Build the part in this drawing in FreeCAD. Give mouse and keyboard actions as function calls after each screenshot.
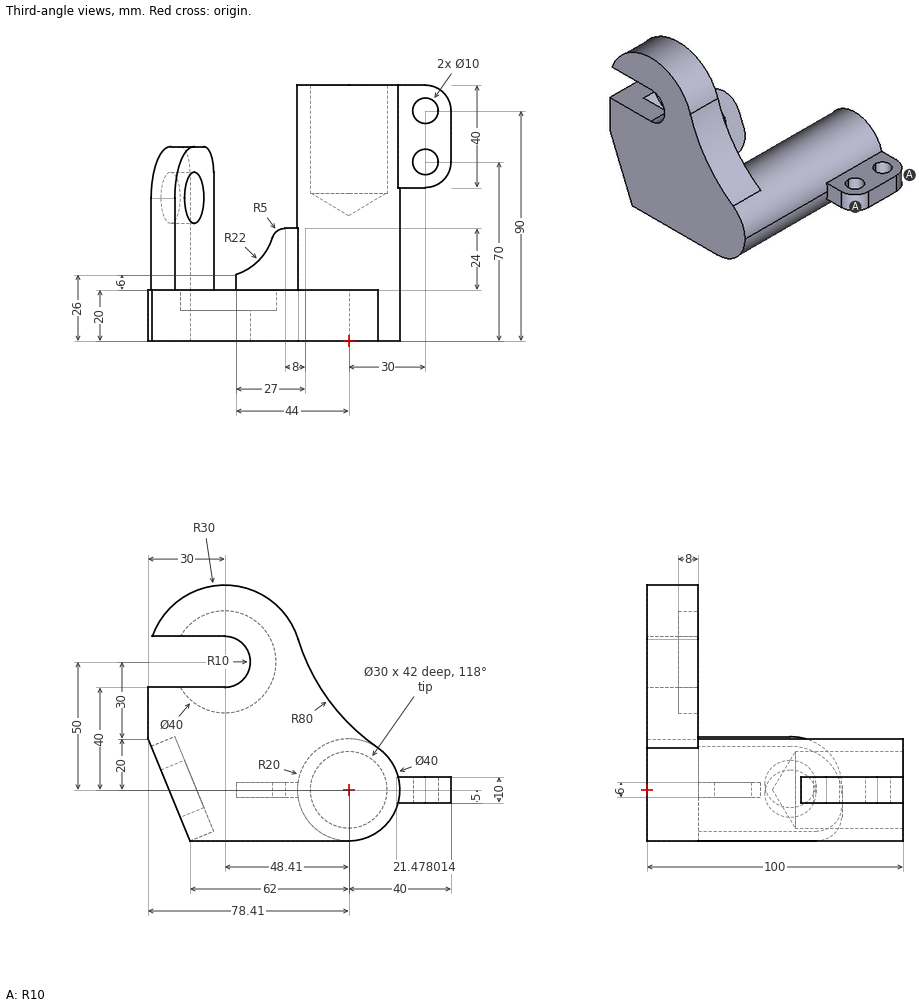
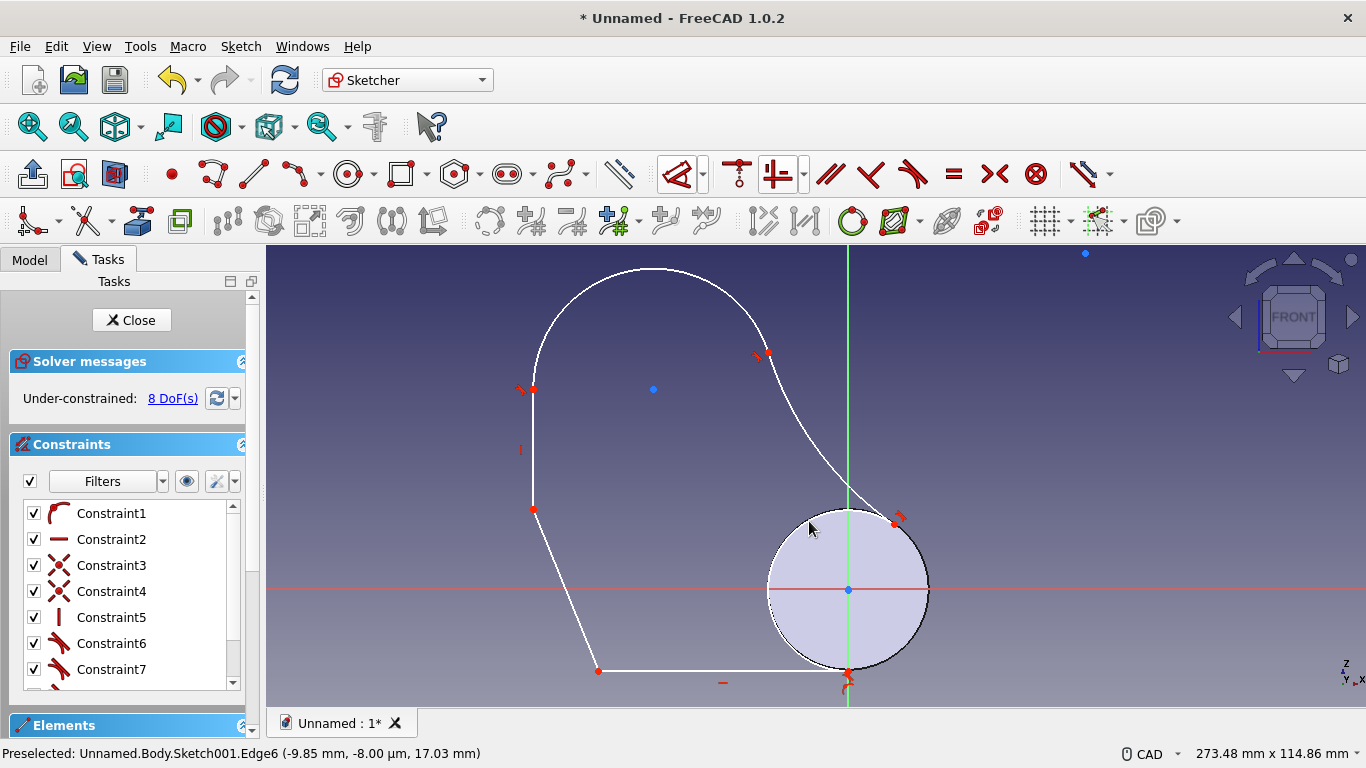
click(848, 591)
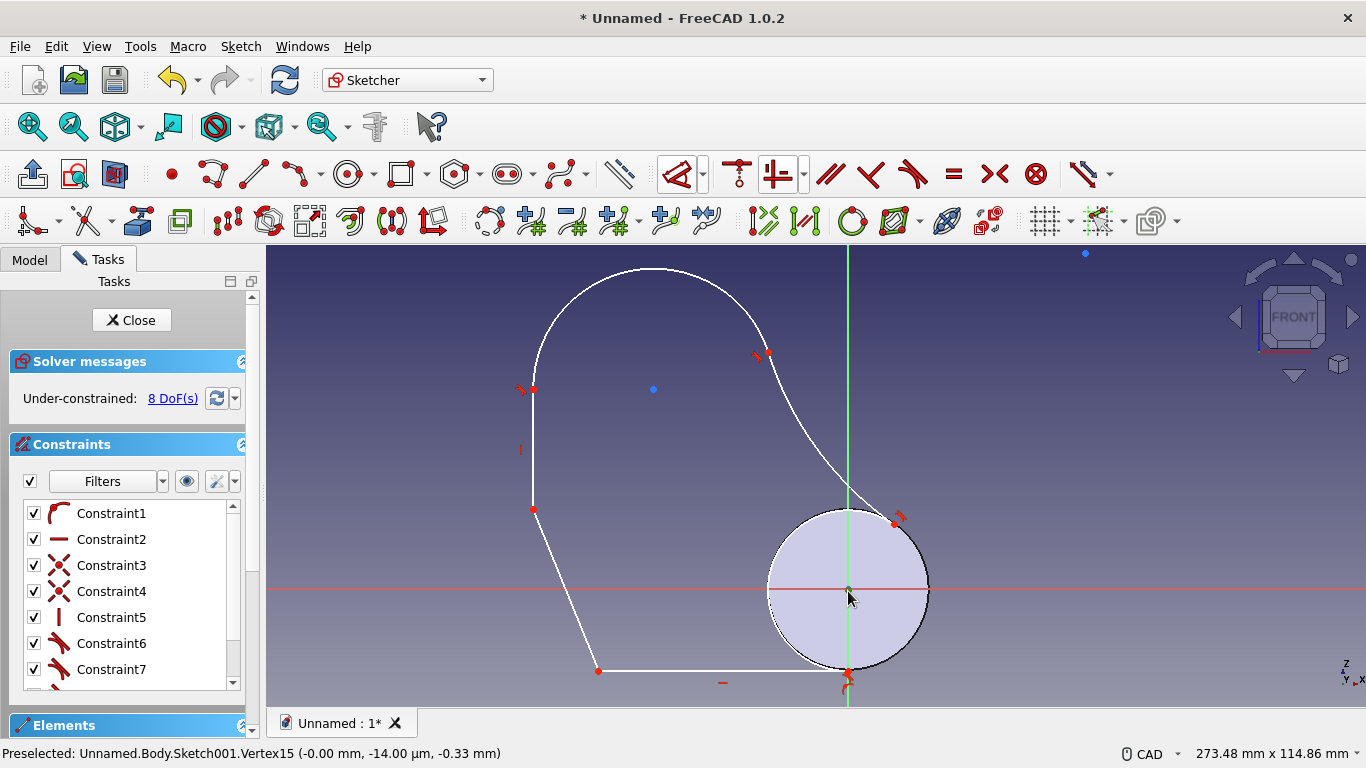
click(359, 589)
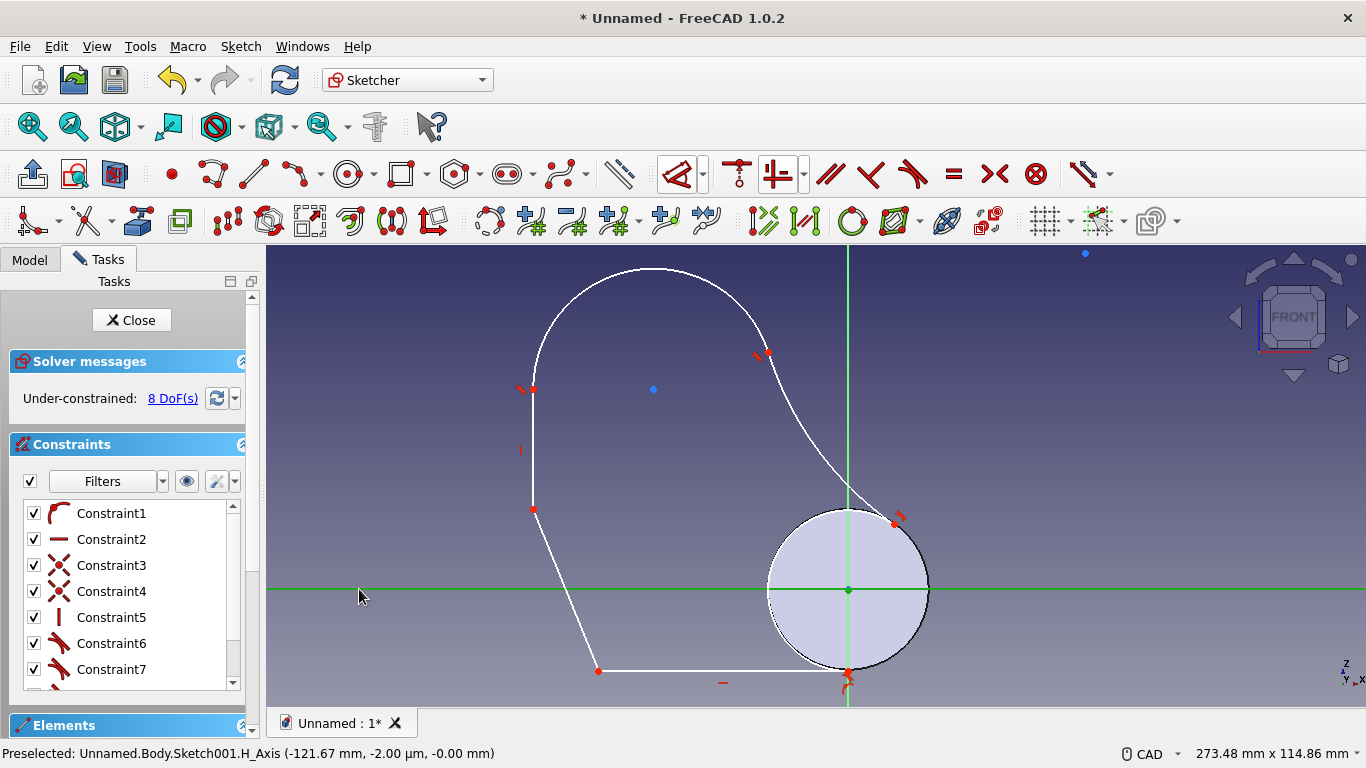
key(c)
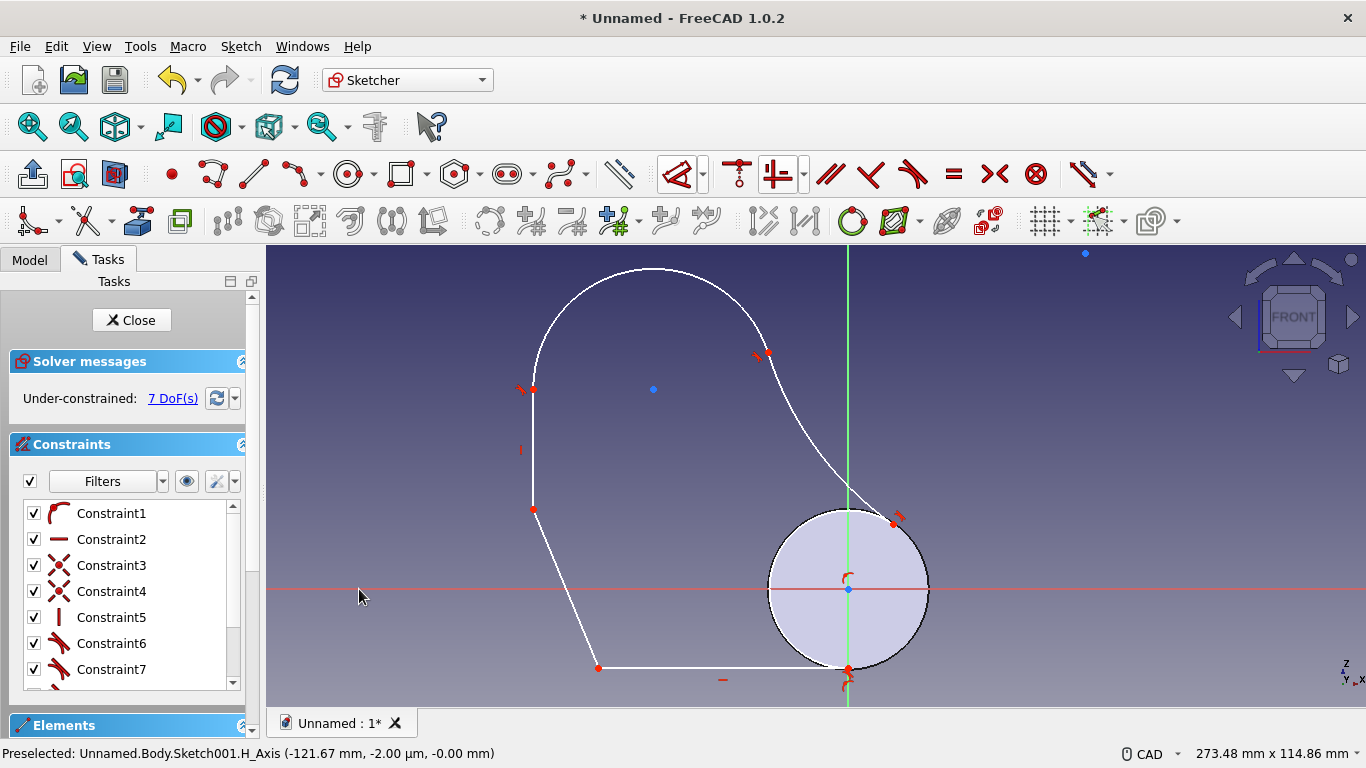
key(d)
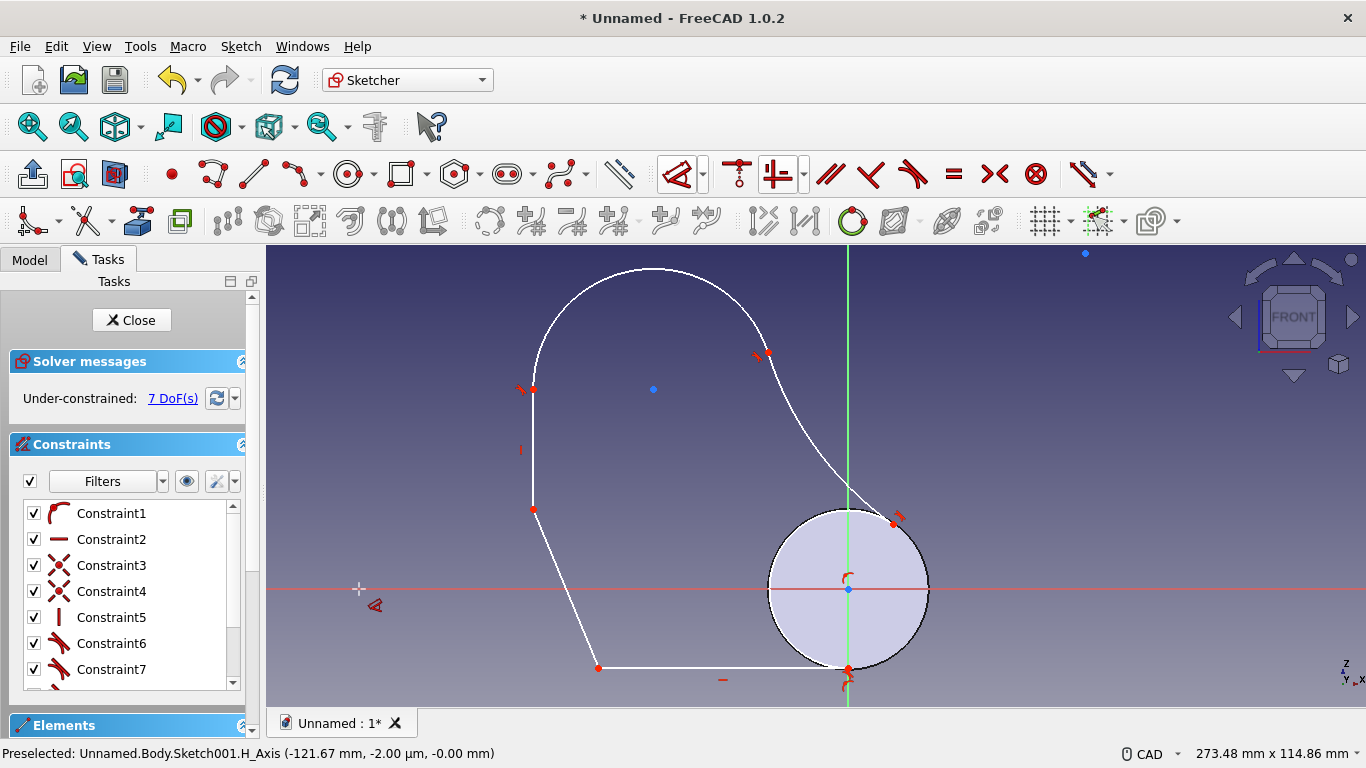
click(702, 279)
click(774, 296)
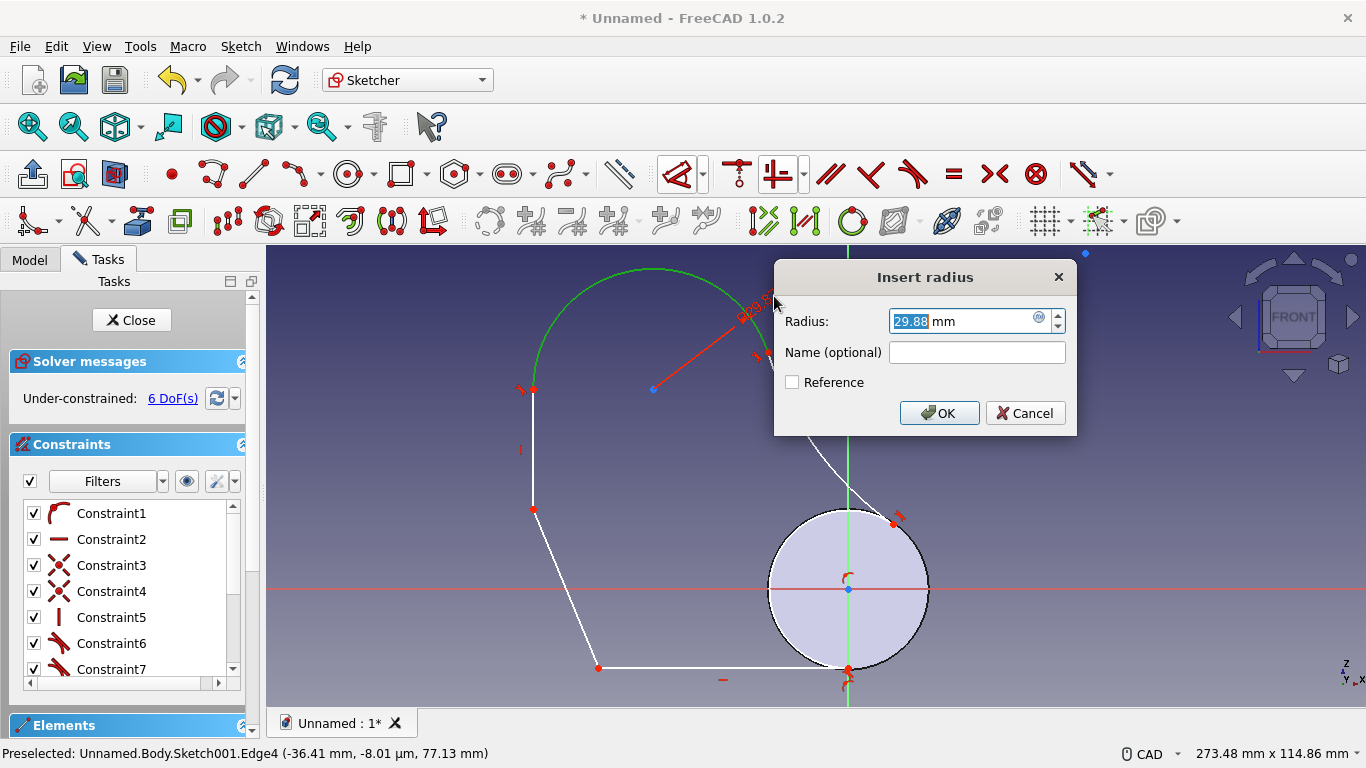
text(30)
key(Return)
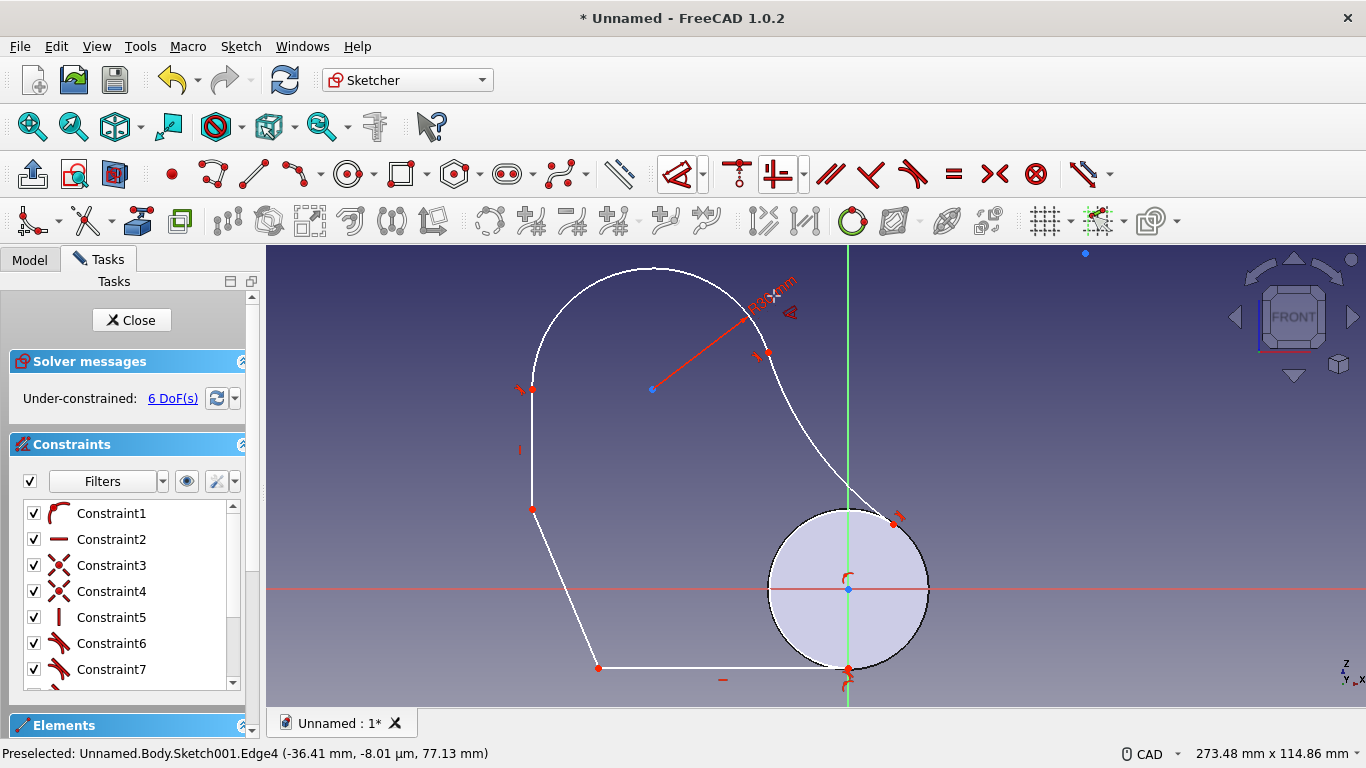
click(794, 413)
click(766, 428)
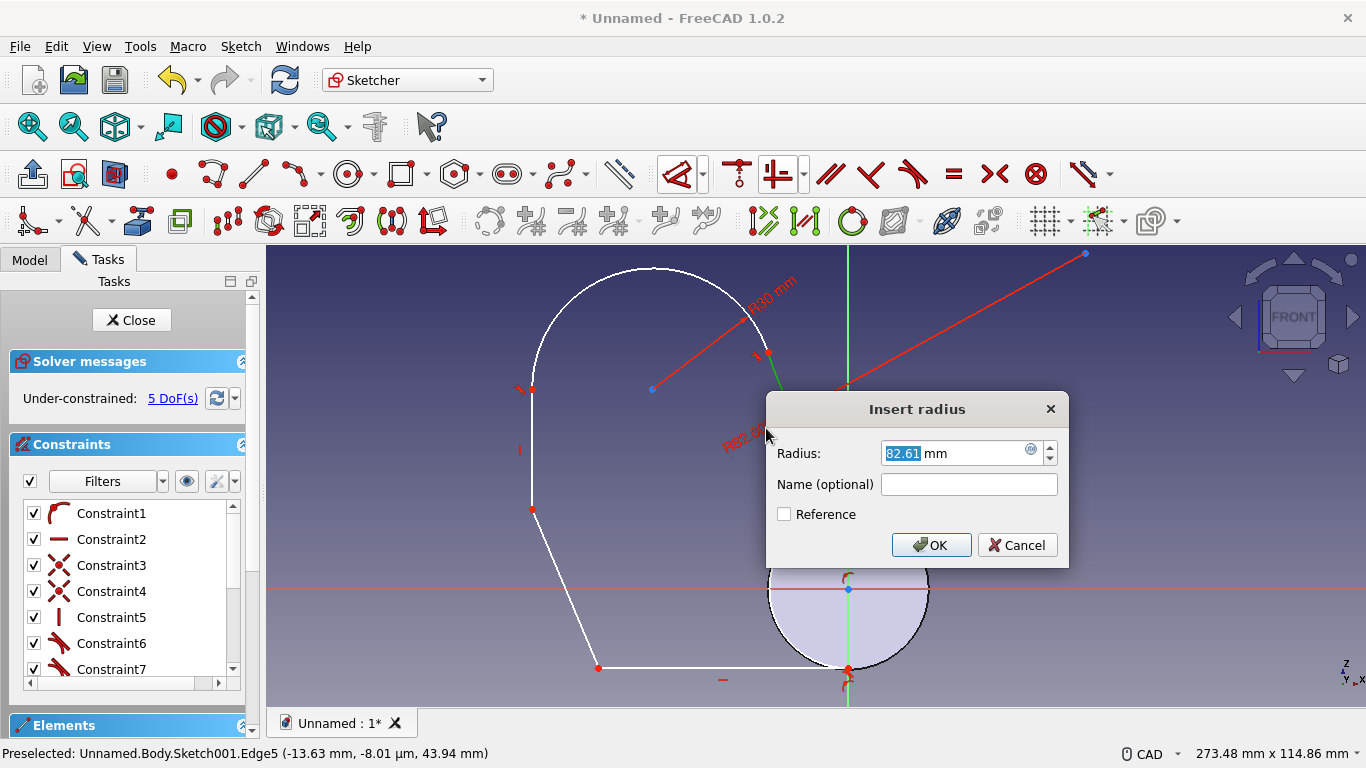
text(80)
key(Return)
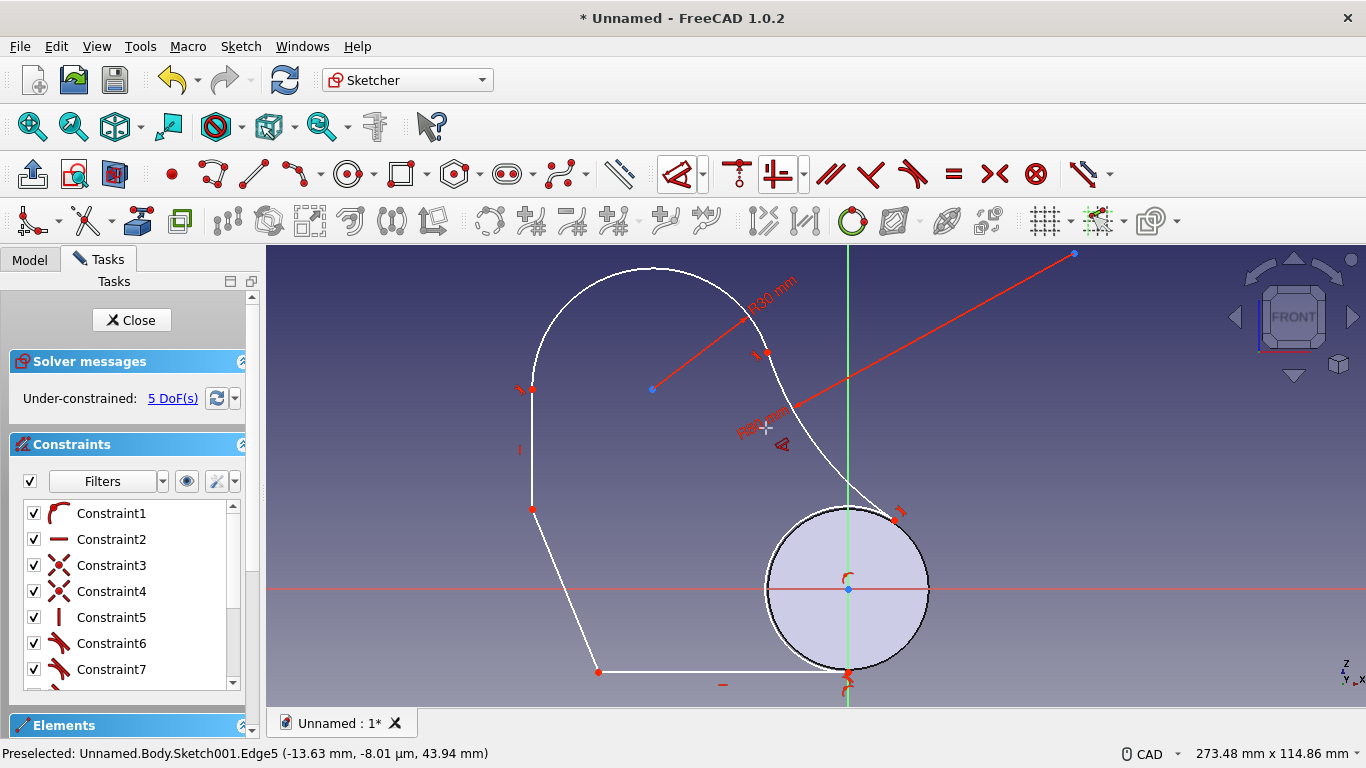
click(806, 518)
click(790, 490)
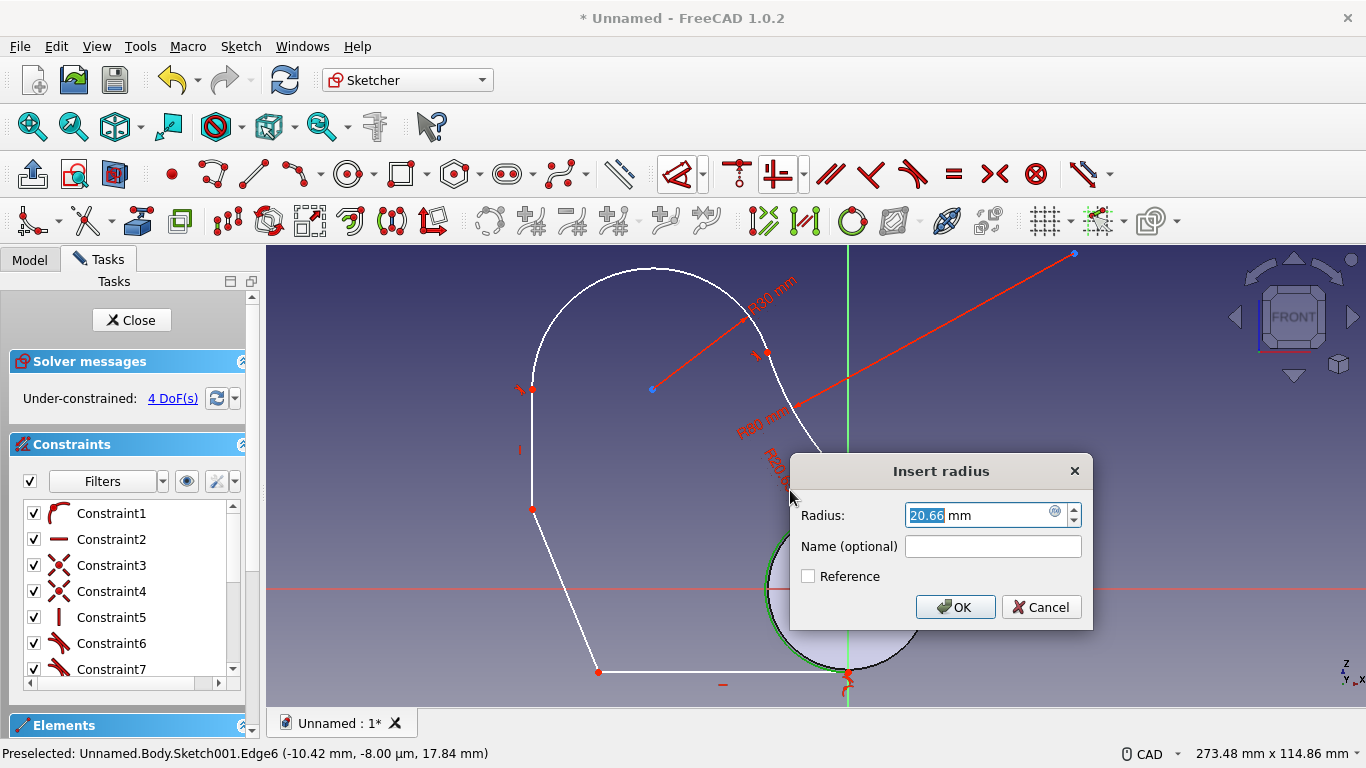
text(20)
key(Return)